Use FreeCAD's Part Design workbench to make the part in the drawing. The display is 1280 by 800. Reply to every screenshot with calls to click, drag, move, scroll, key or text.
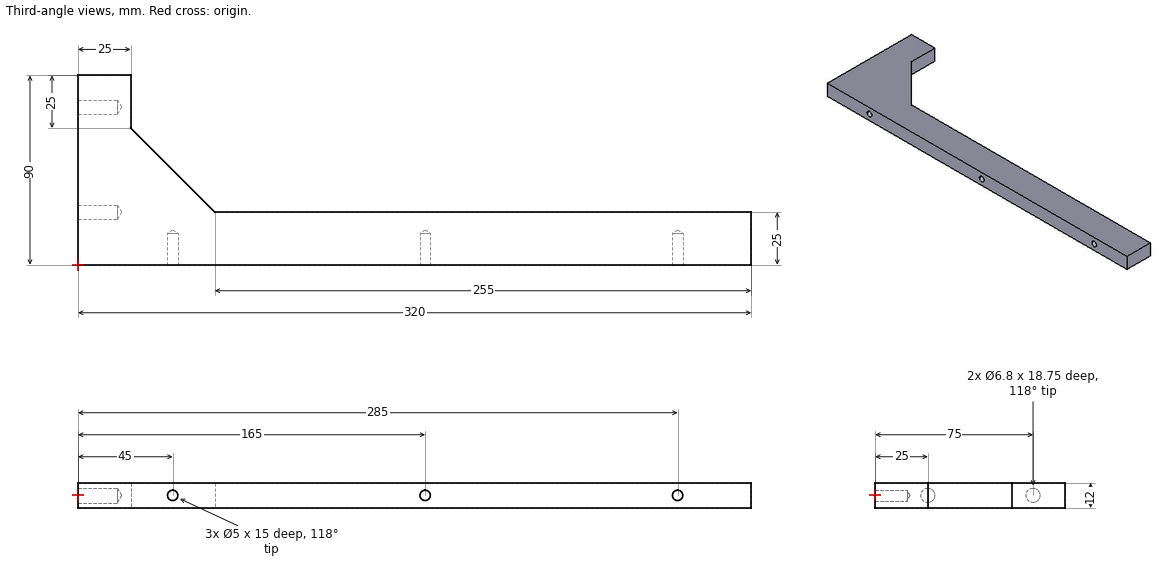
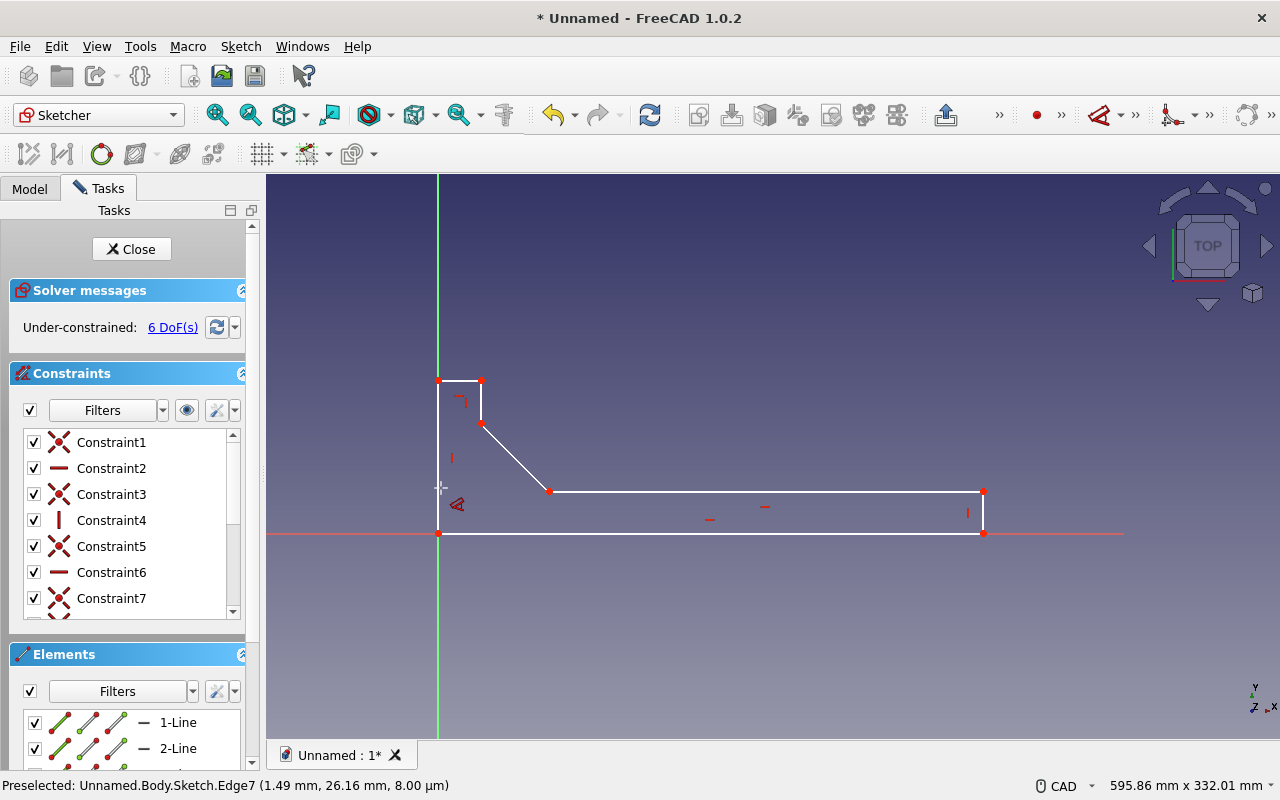
click(983, 521)
click(1017, 513)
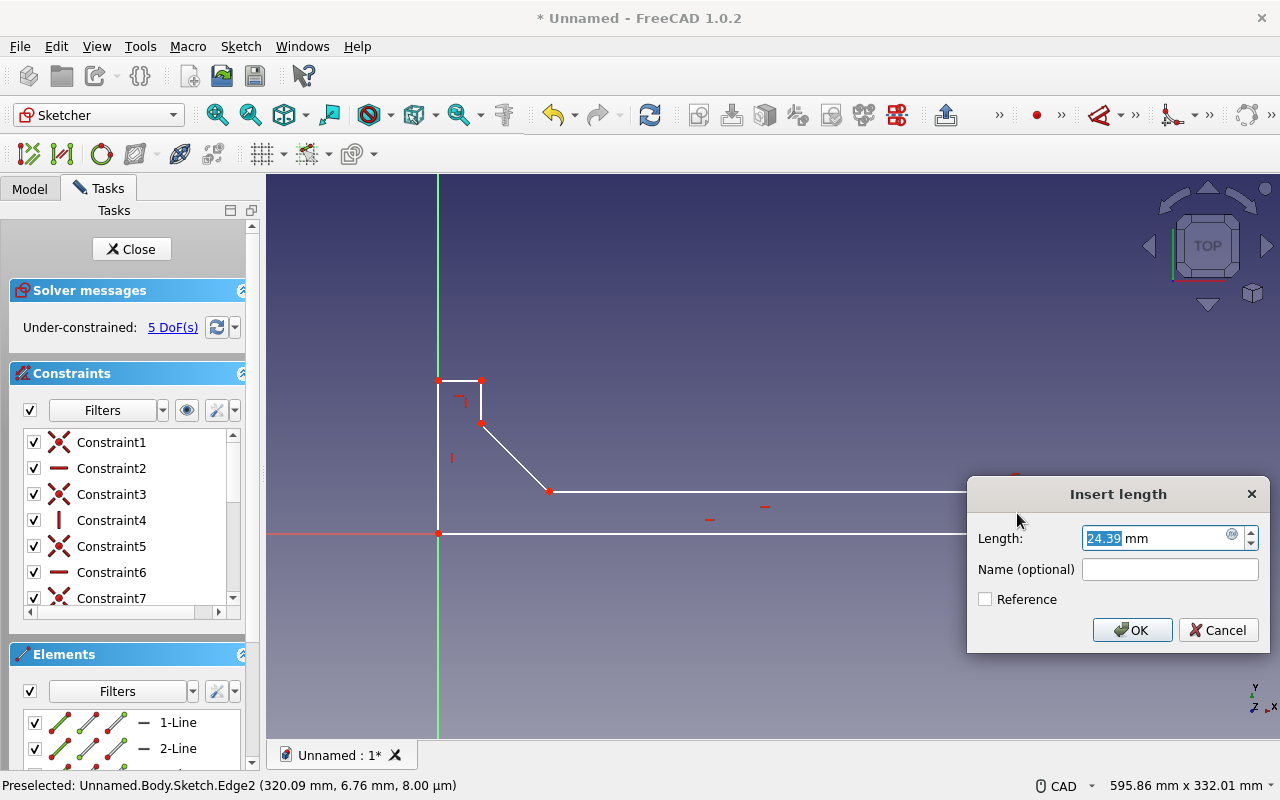
text(25)
key(Return)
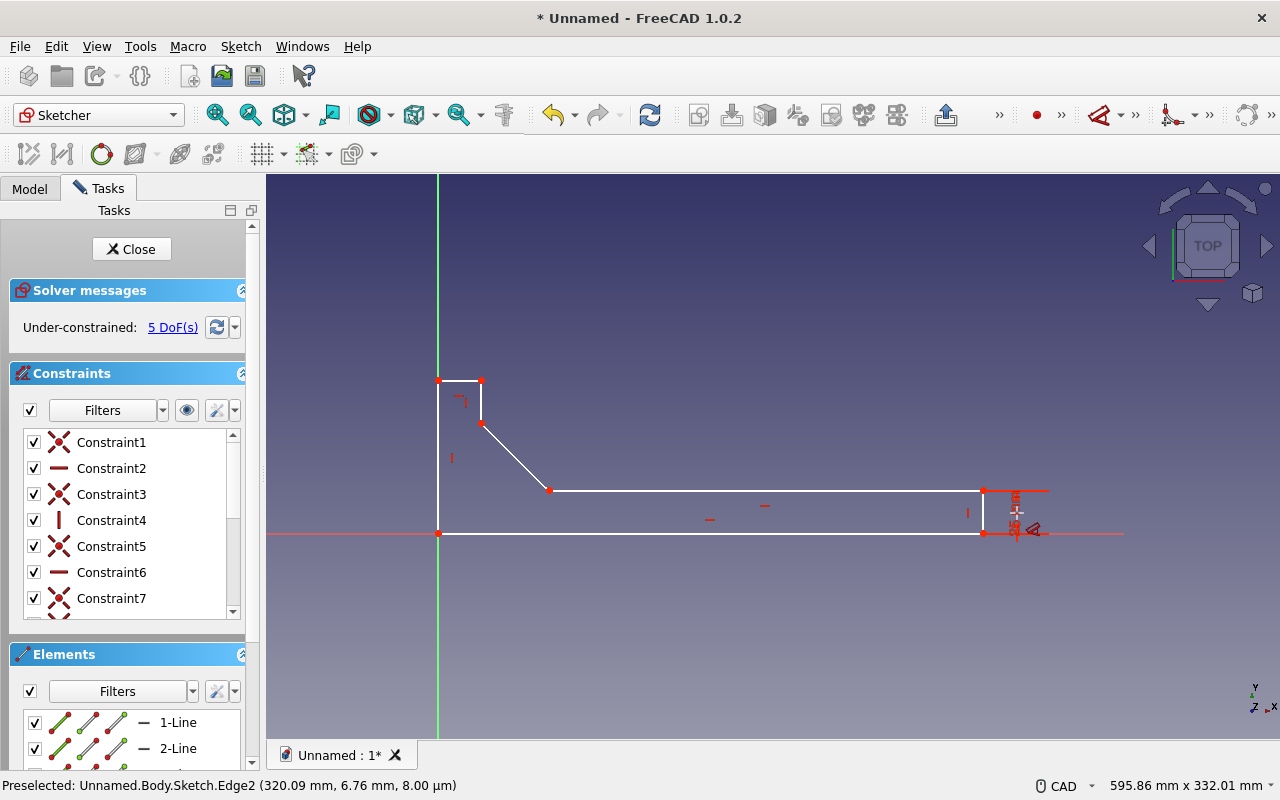
click(481, 411)
click(515, 403)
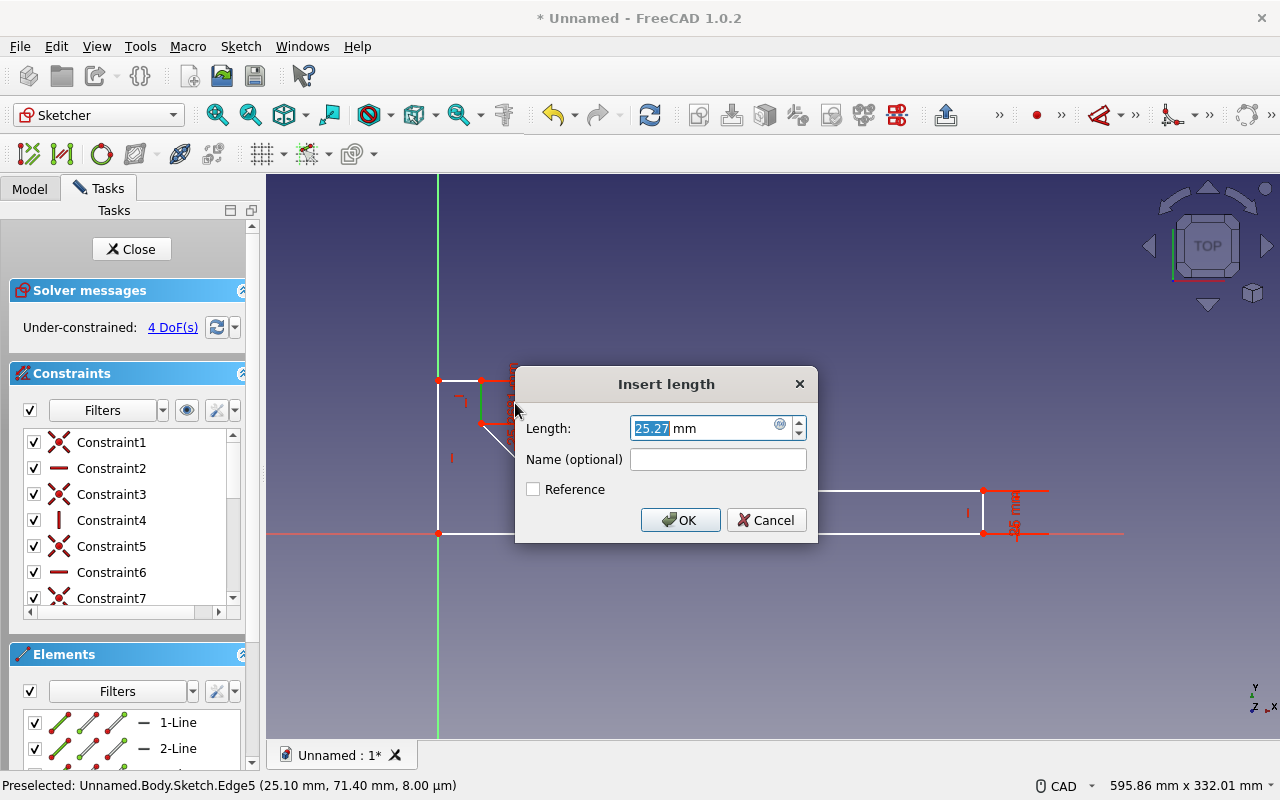
text(25)
key(Return)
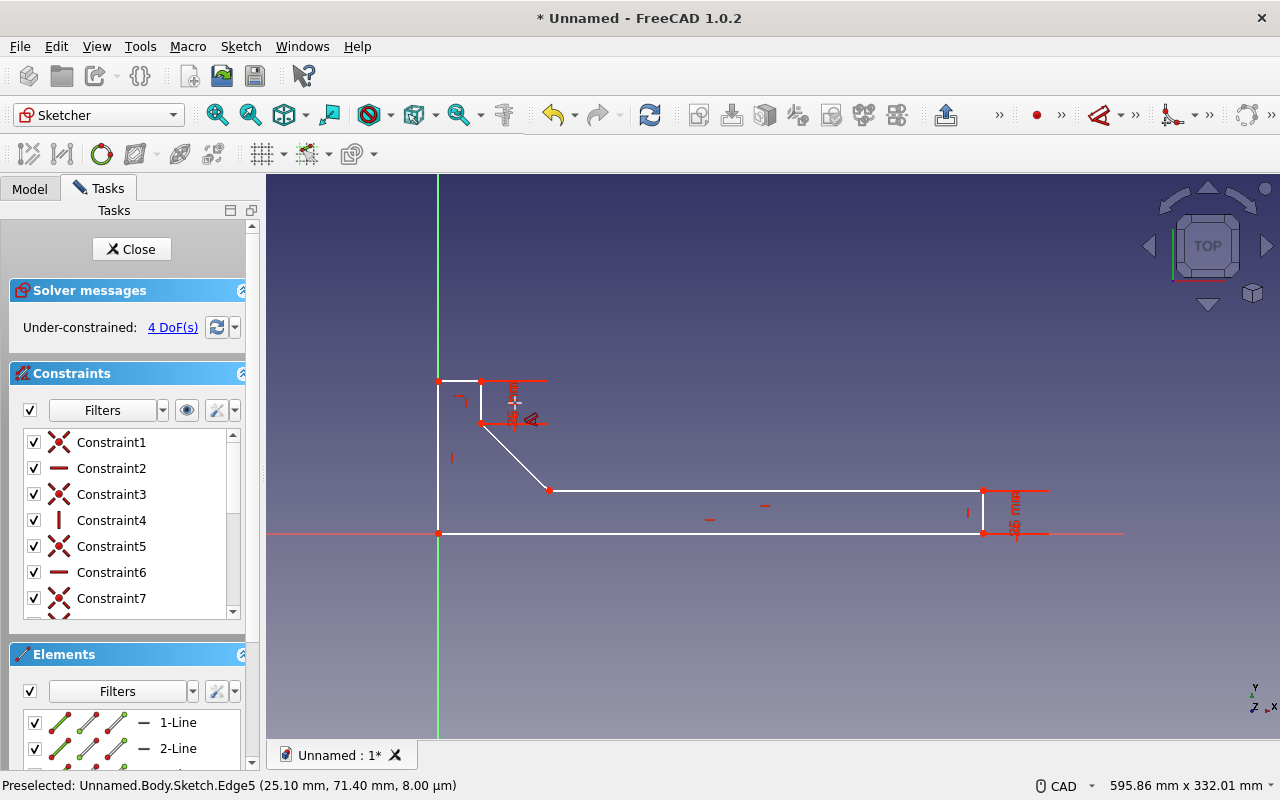
click(468, 381)
click(460, 347)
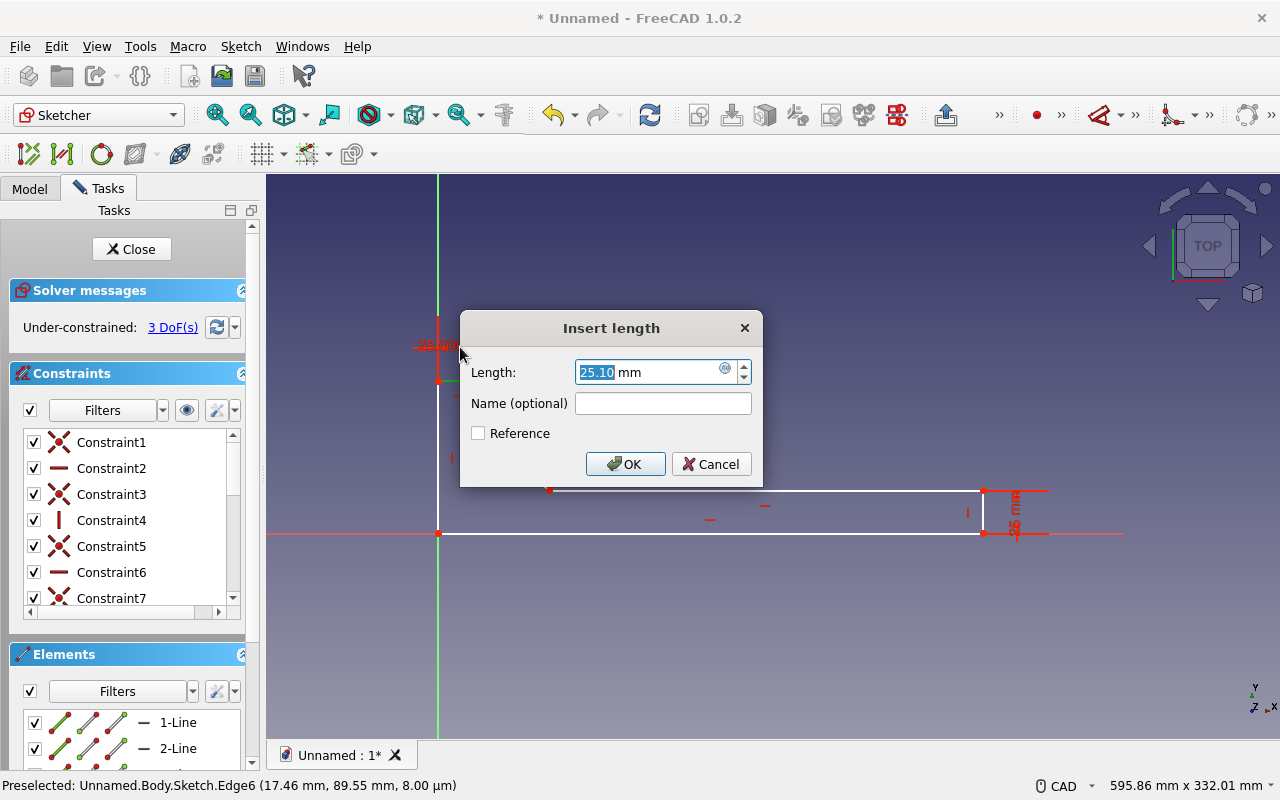
text(25)
key(Return)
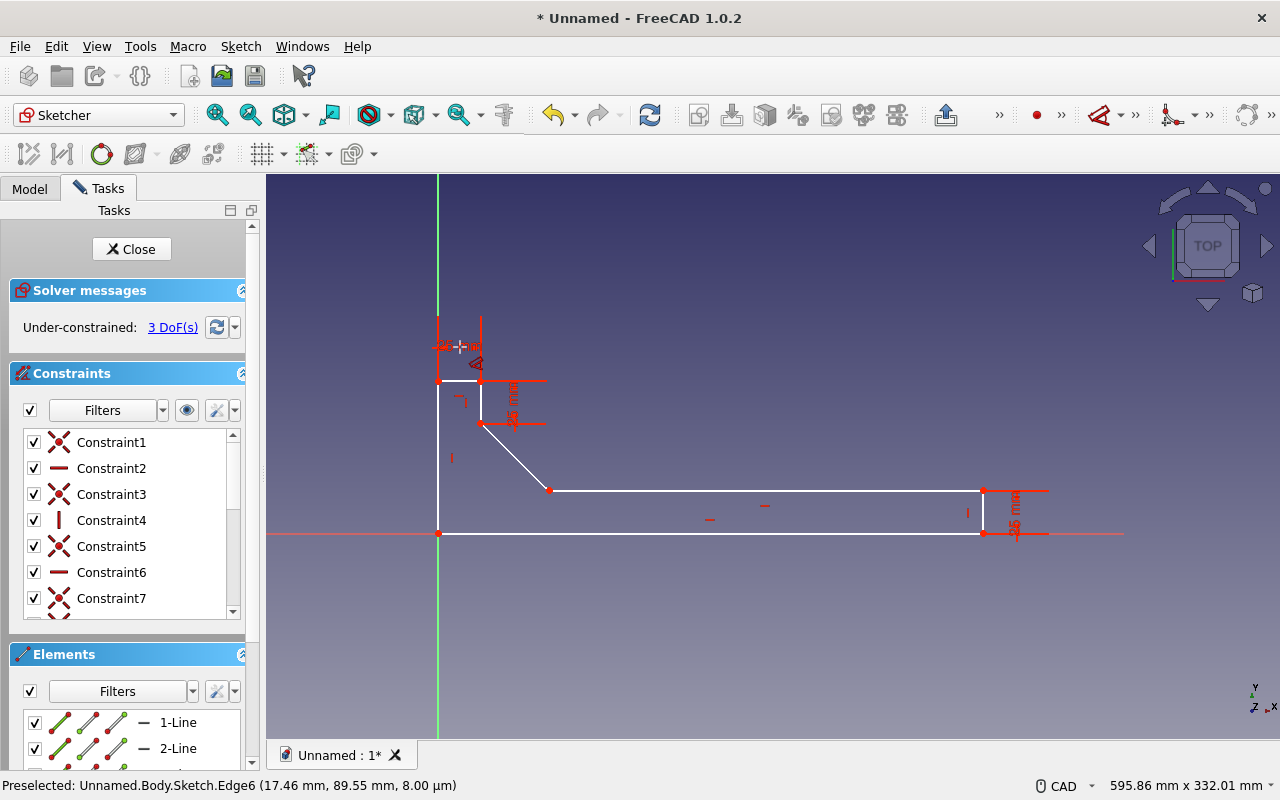
click(438, 427)
click(404, 457)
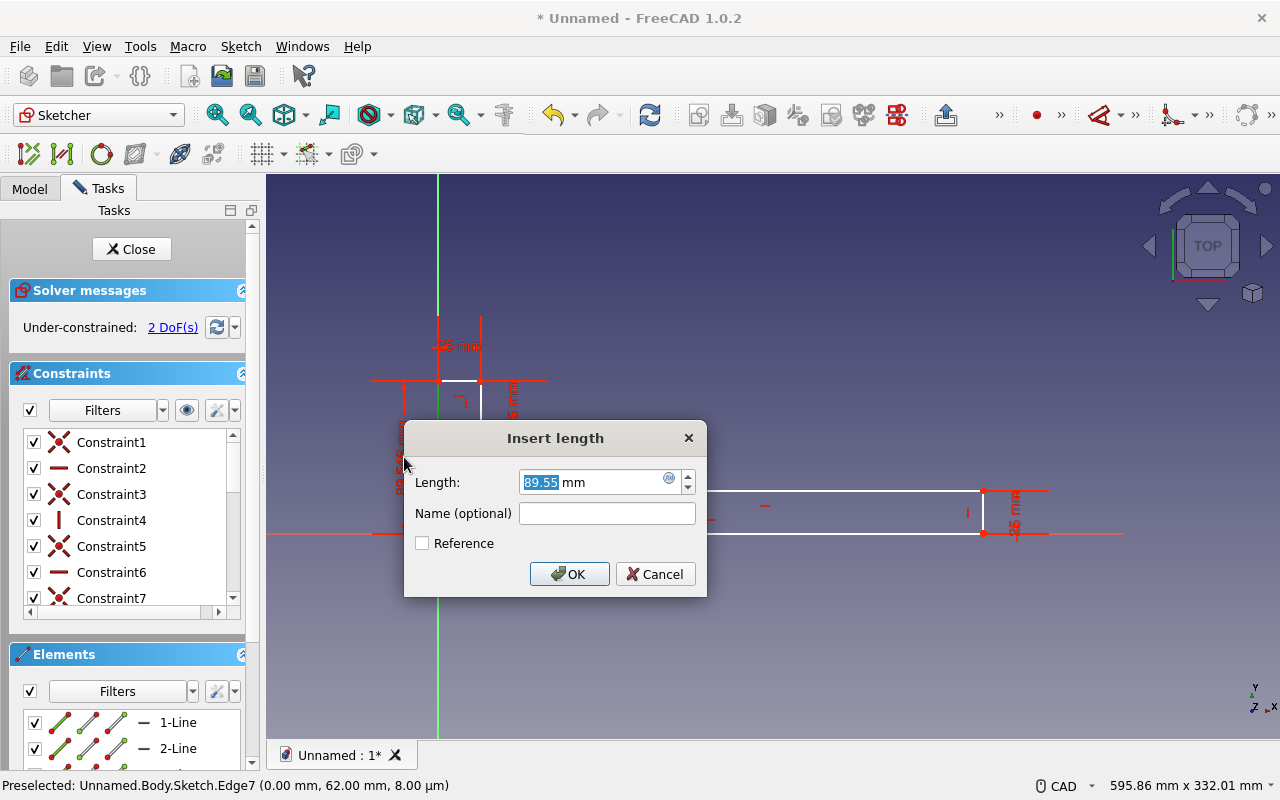
text(90)
key(Return)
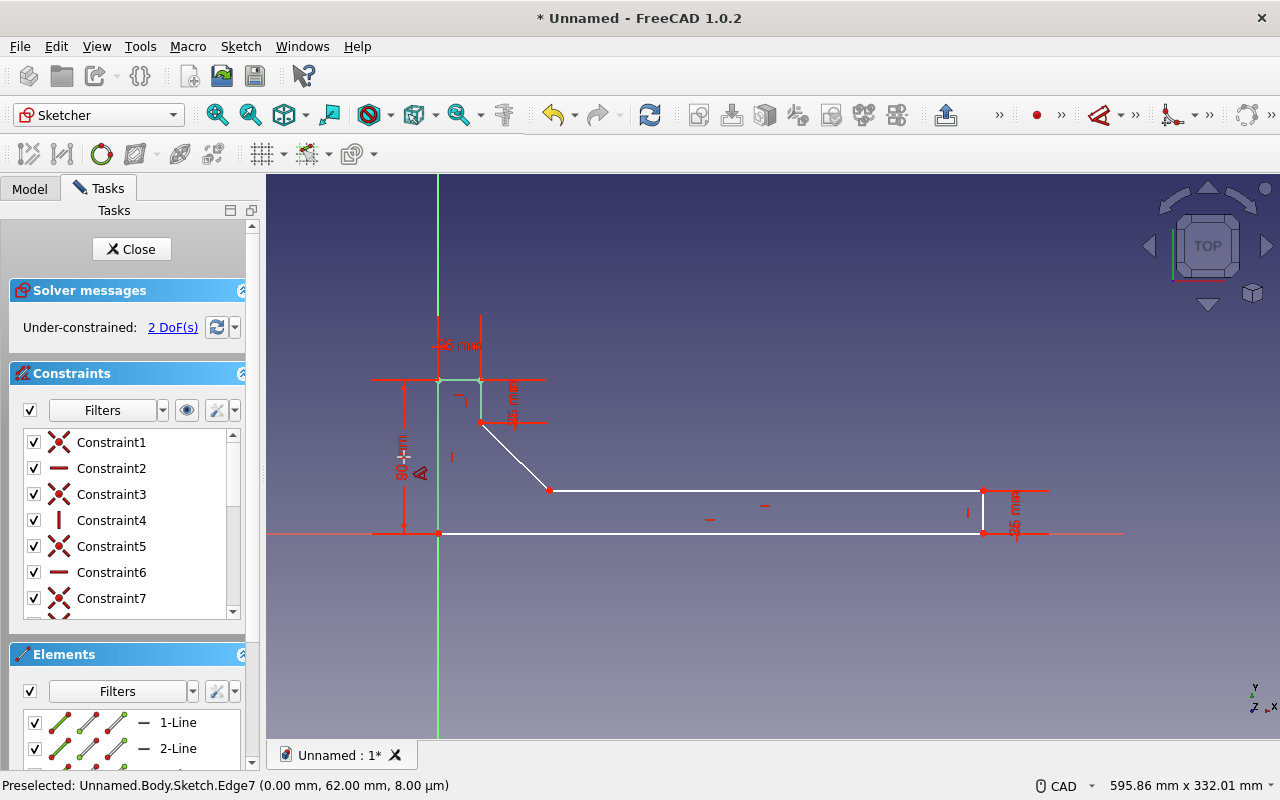
click(602, 534)
click(711, 568)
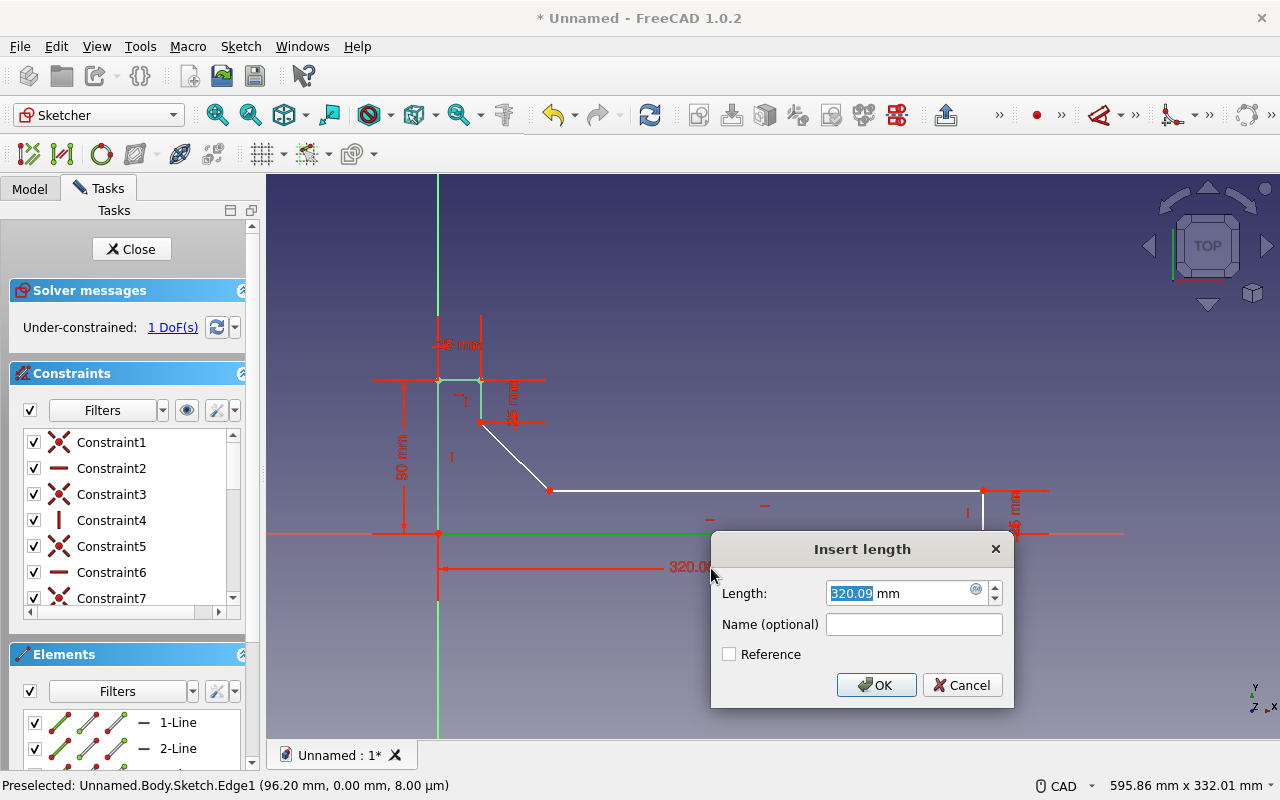
text(320)
key(Return)